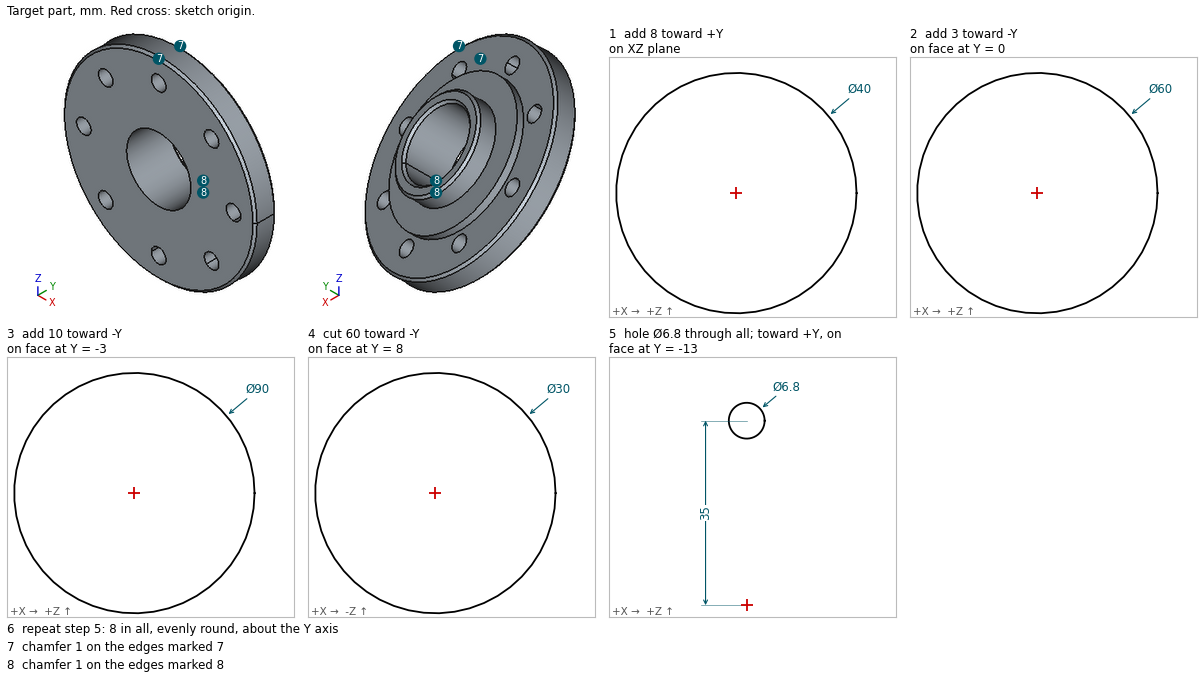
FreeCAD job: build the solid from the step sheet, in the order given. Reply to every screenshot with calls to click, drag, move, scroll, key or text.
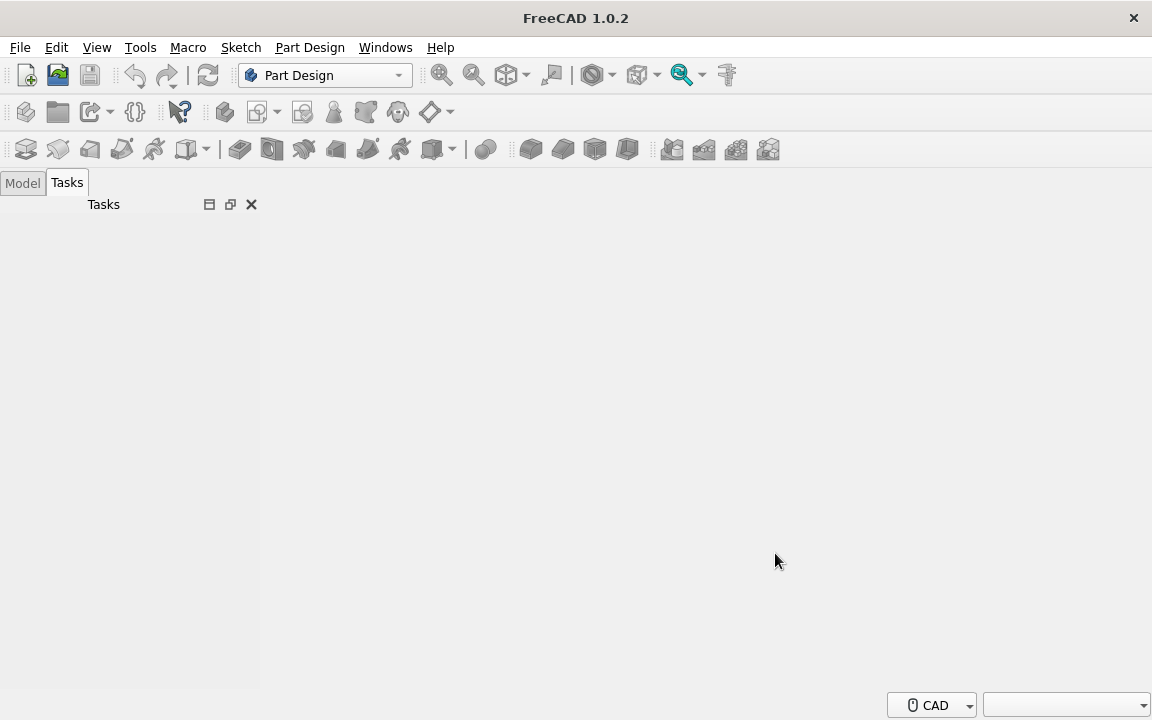
click(26, 76)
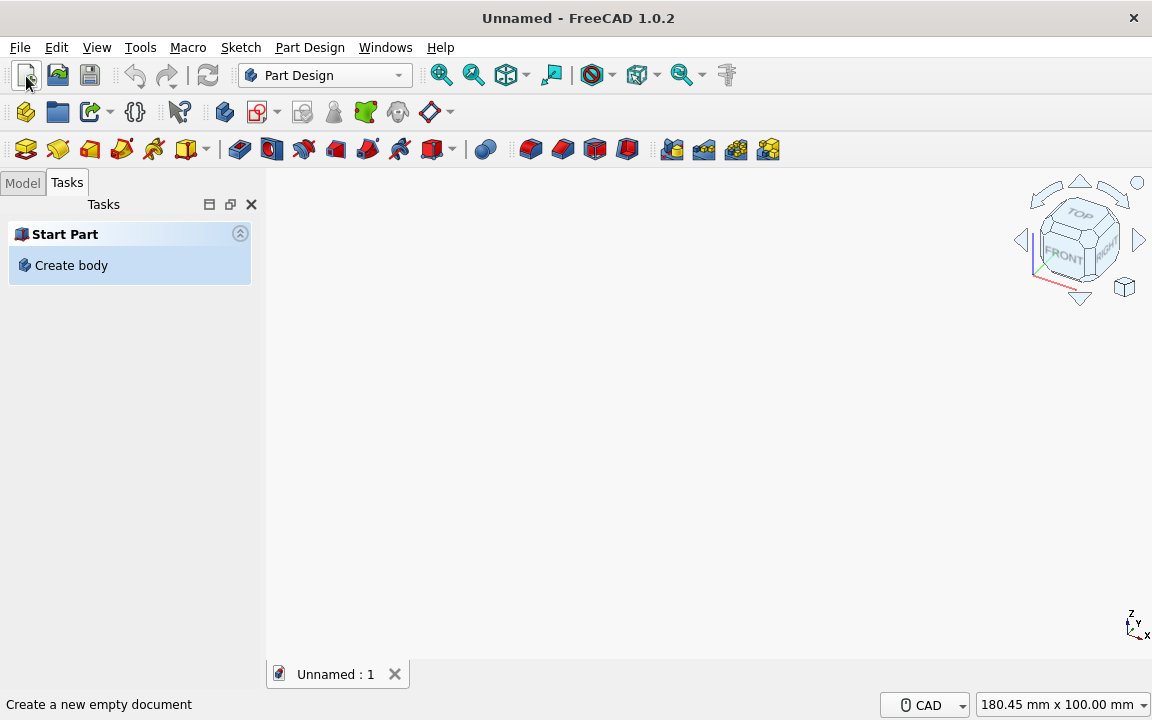
click(258, 112)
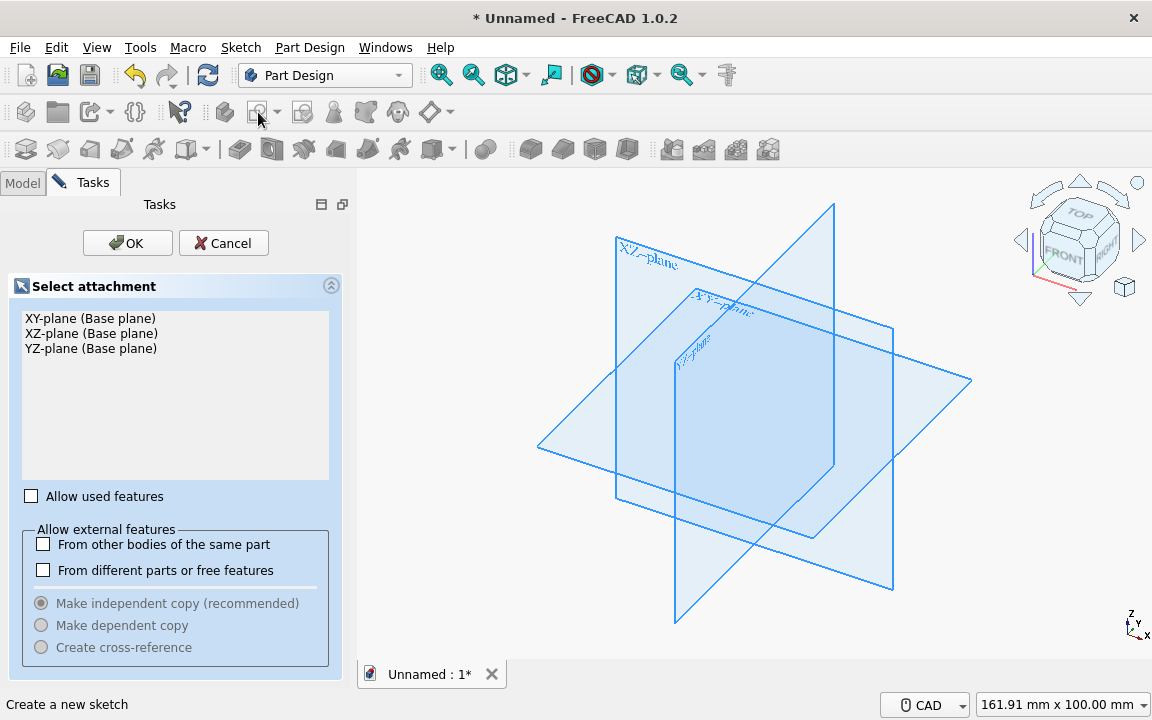
click(82, 334)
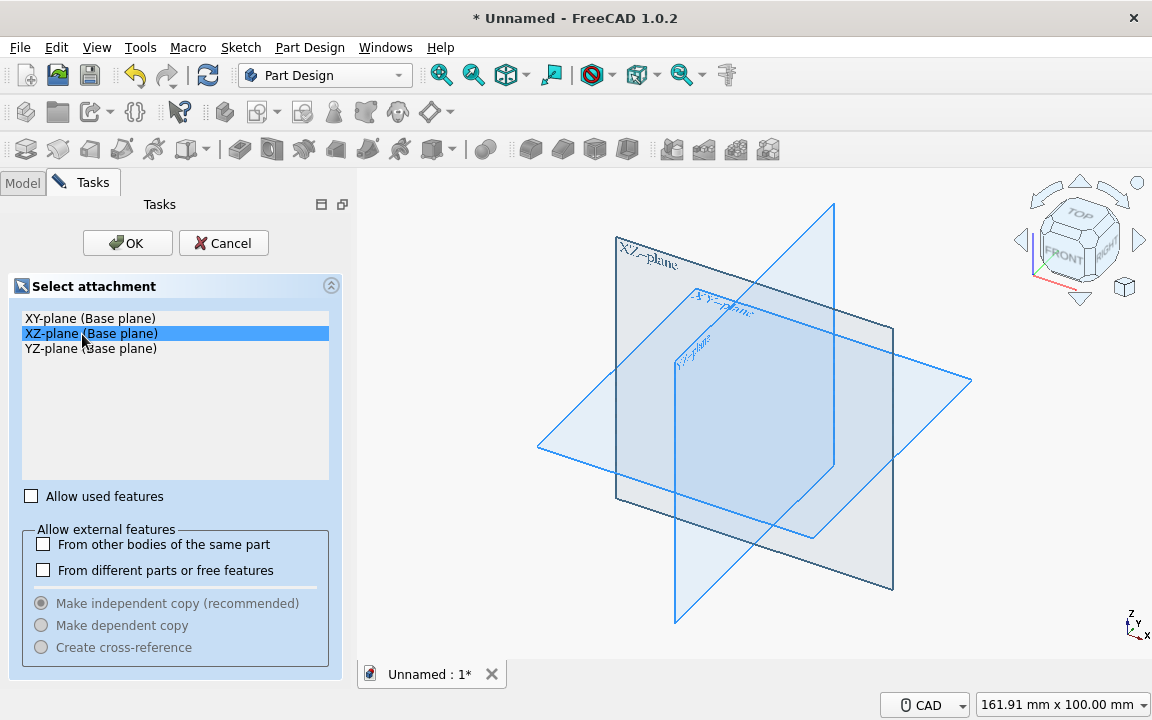
click(128, 243)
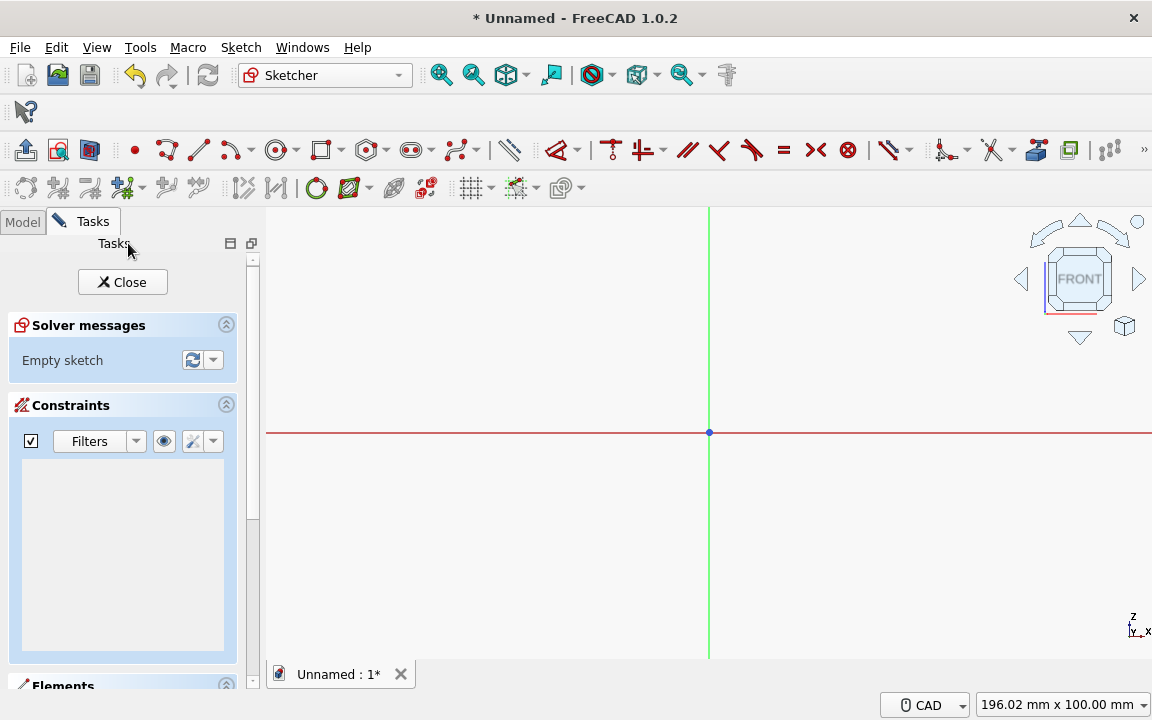
scroll(848, 433, up, 2)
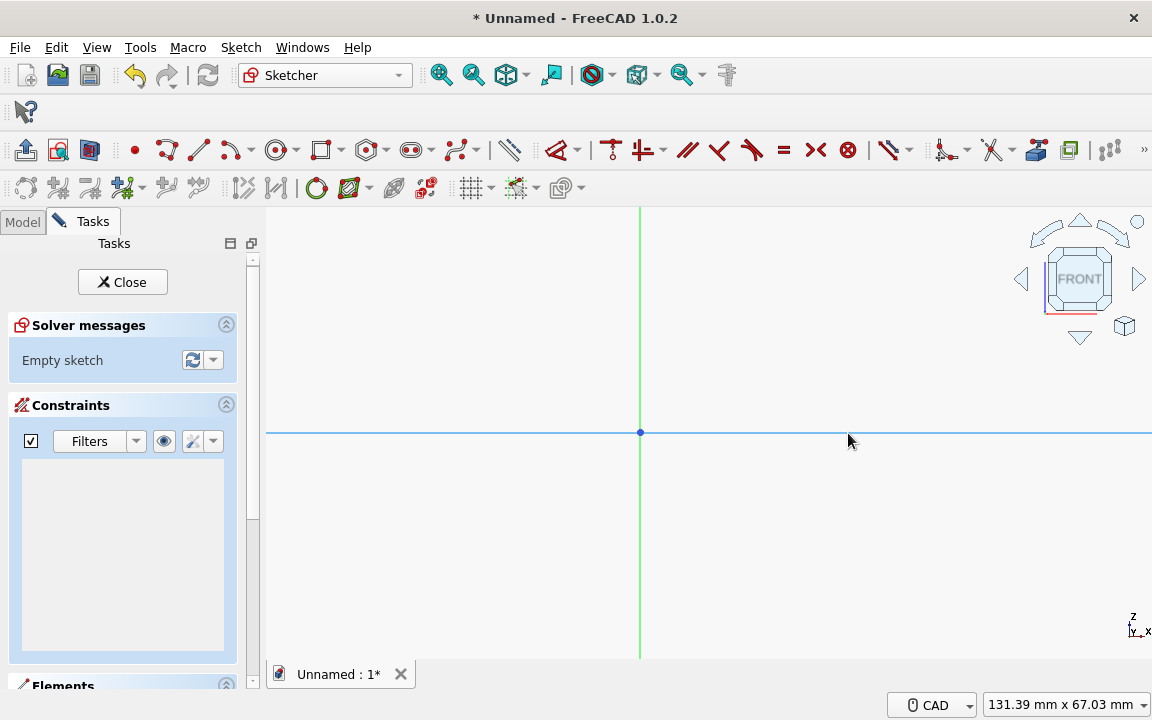
click(276, 150)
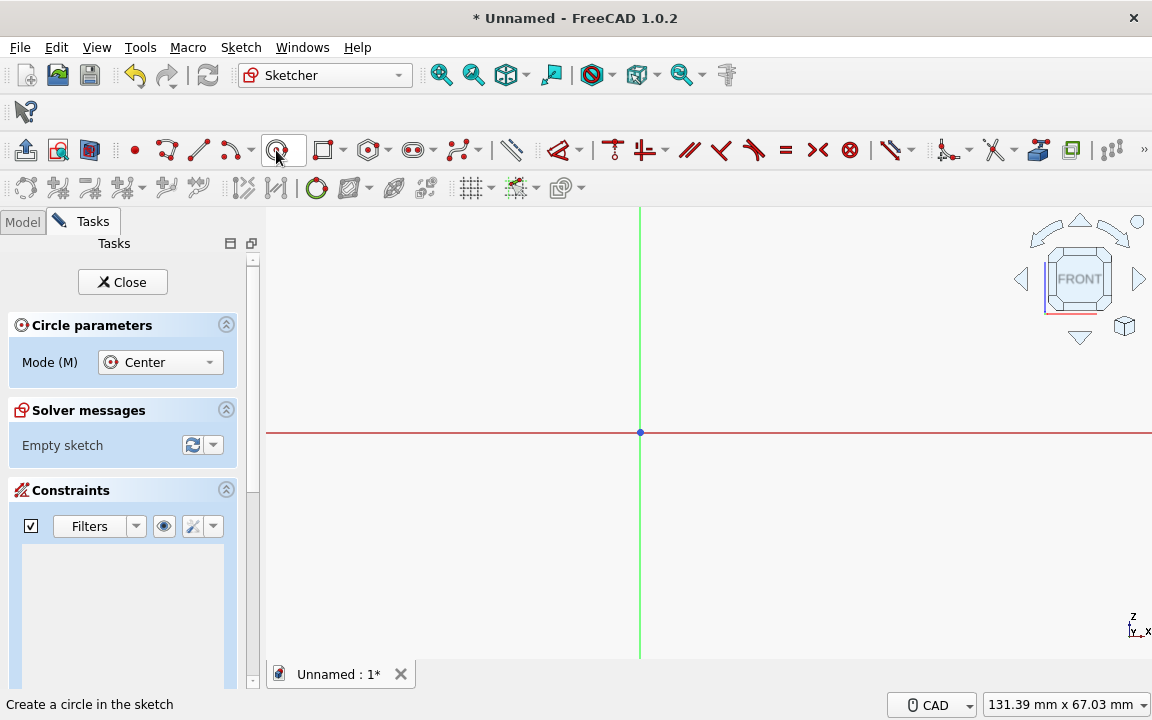
click(640, 433)
move(736, 337)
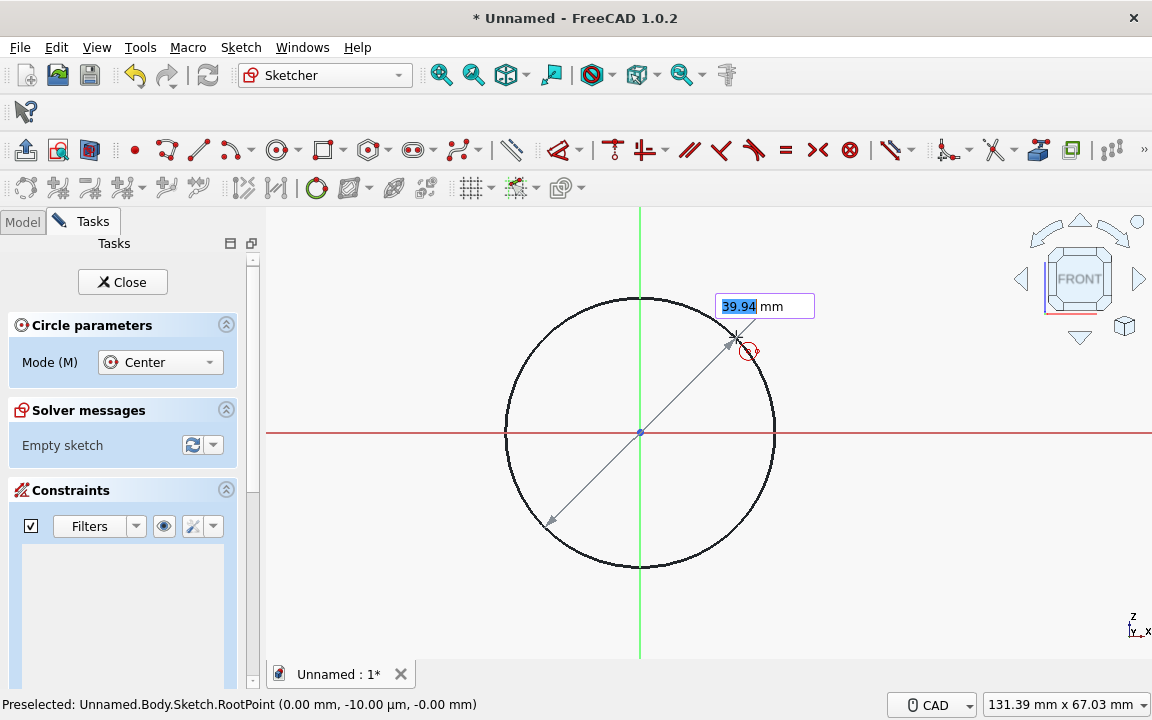
text(40)
key(Return)
key(Escape)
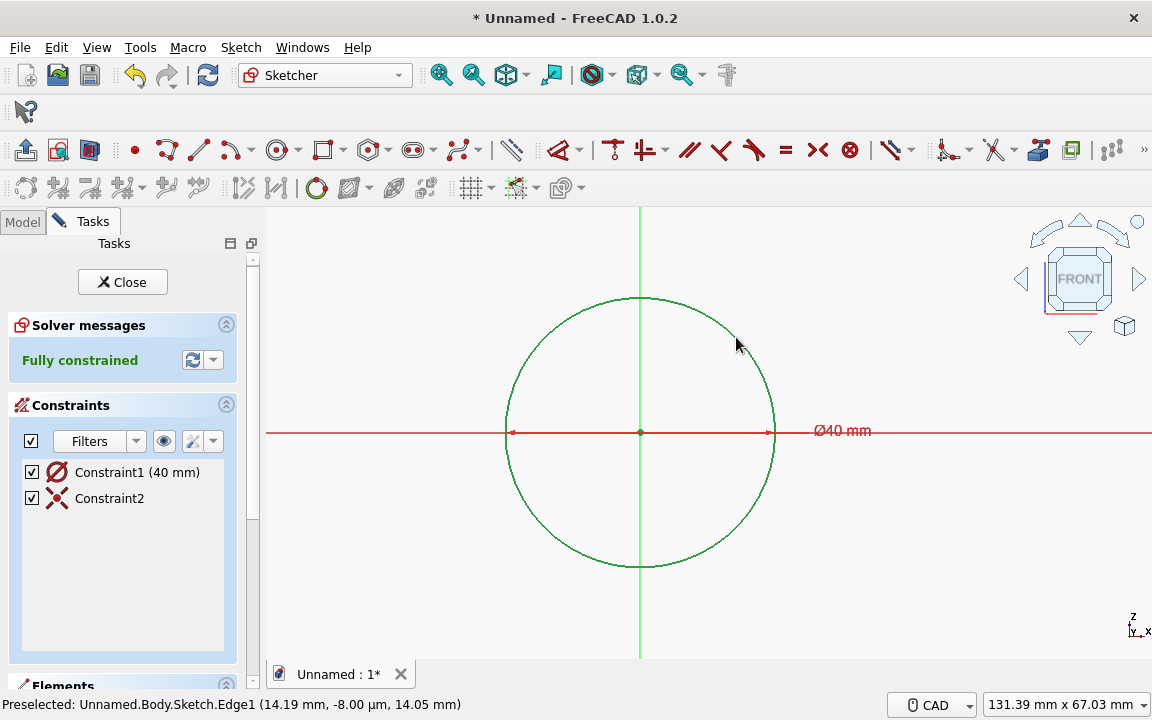
click(123, 282)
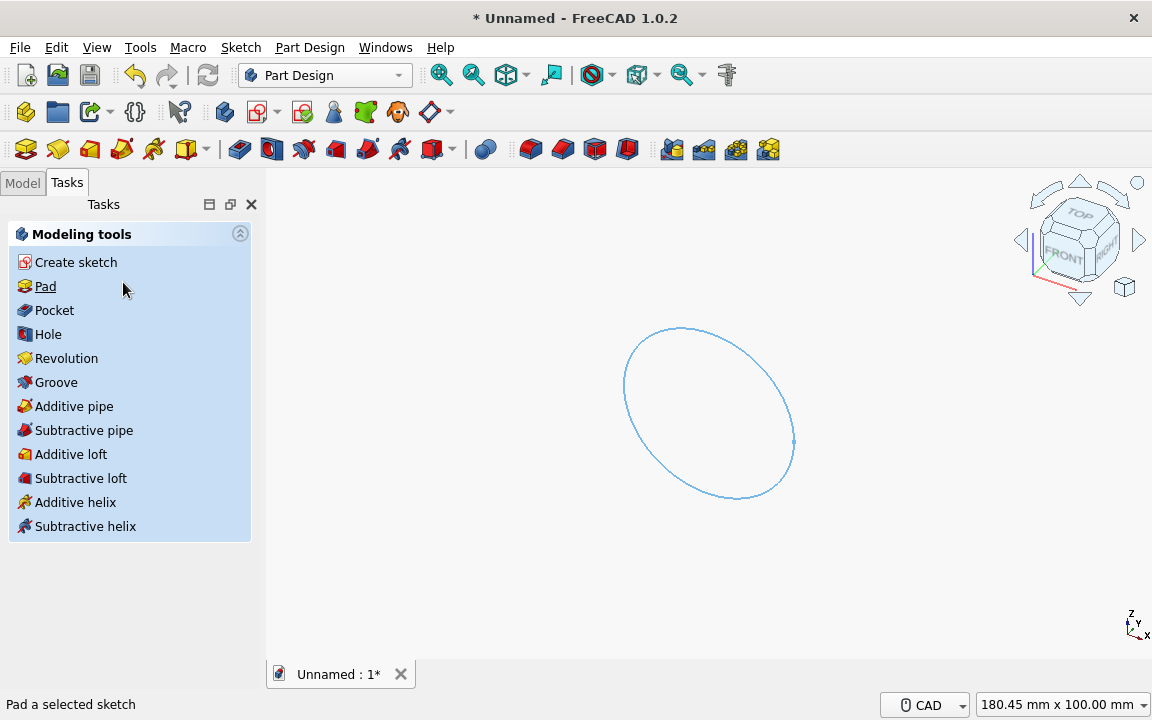
click(26, 150)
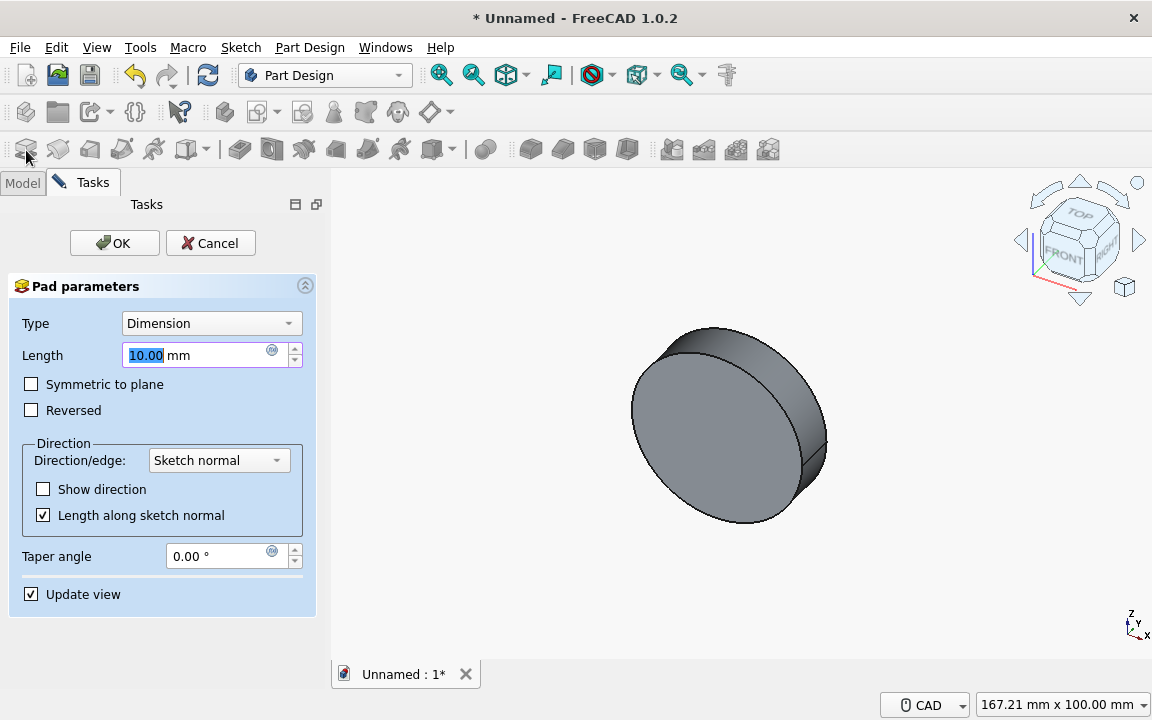
text(8)
key(Tab)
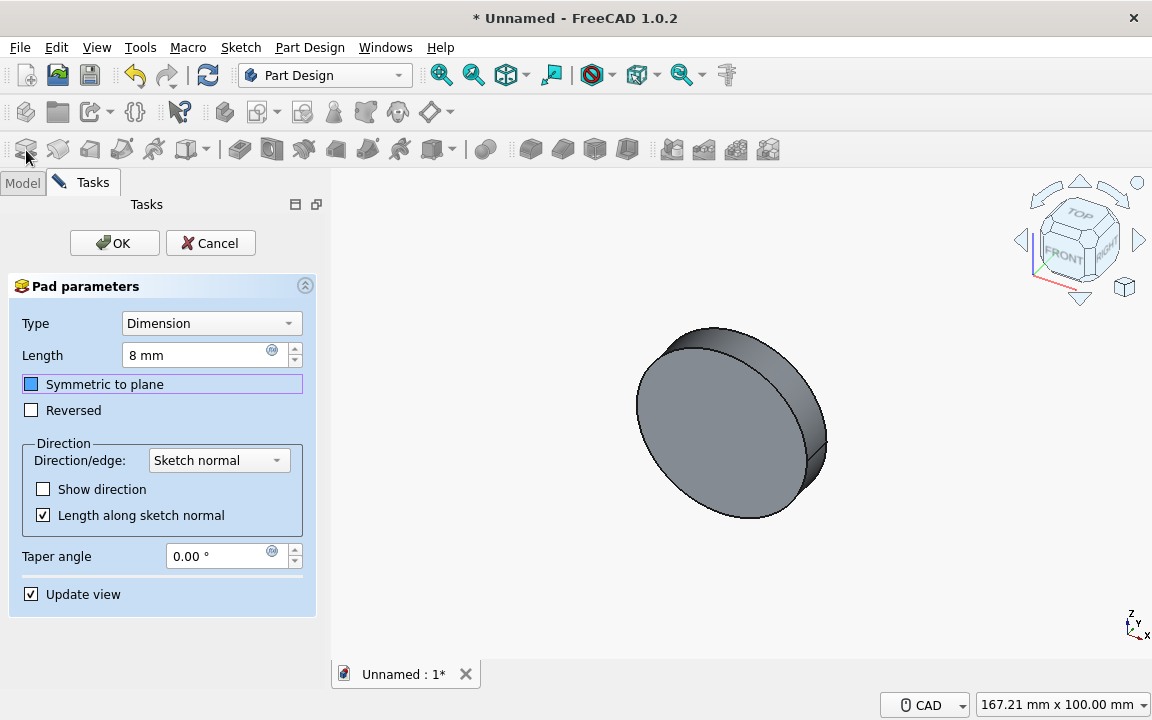
click(30, 410)